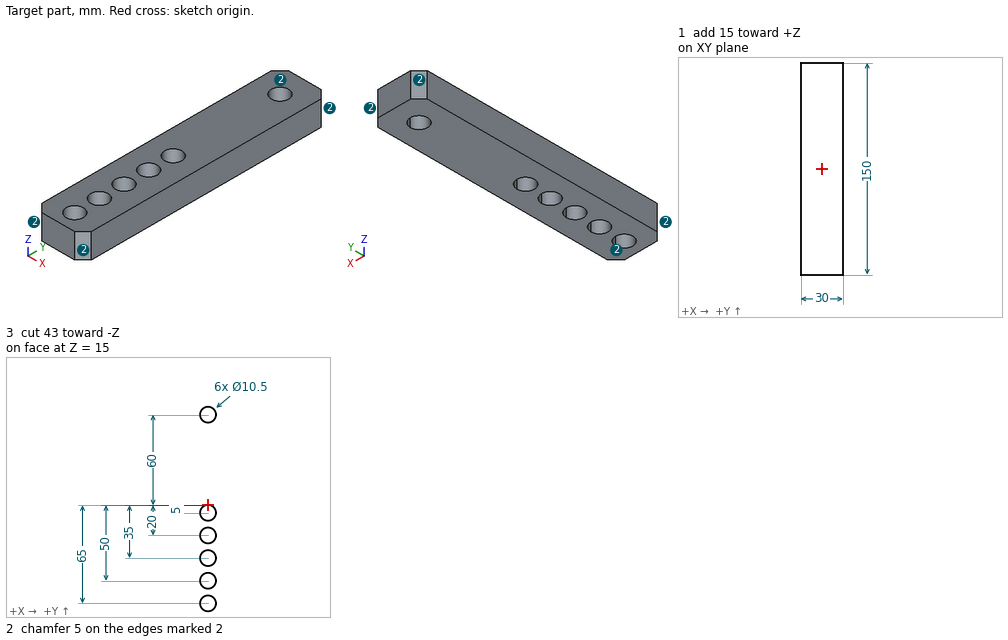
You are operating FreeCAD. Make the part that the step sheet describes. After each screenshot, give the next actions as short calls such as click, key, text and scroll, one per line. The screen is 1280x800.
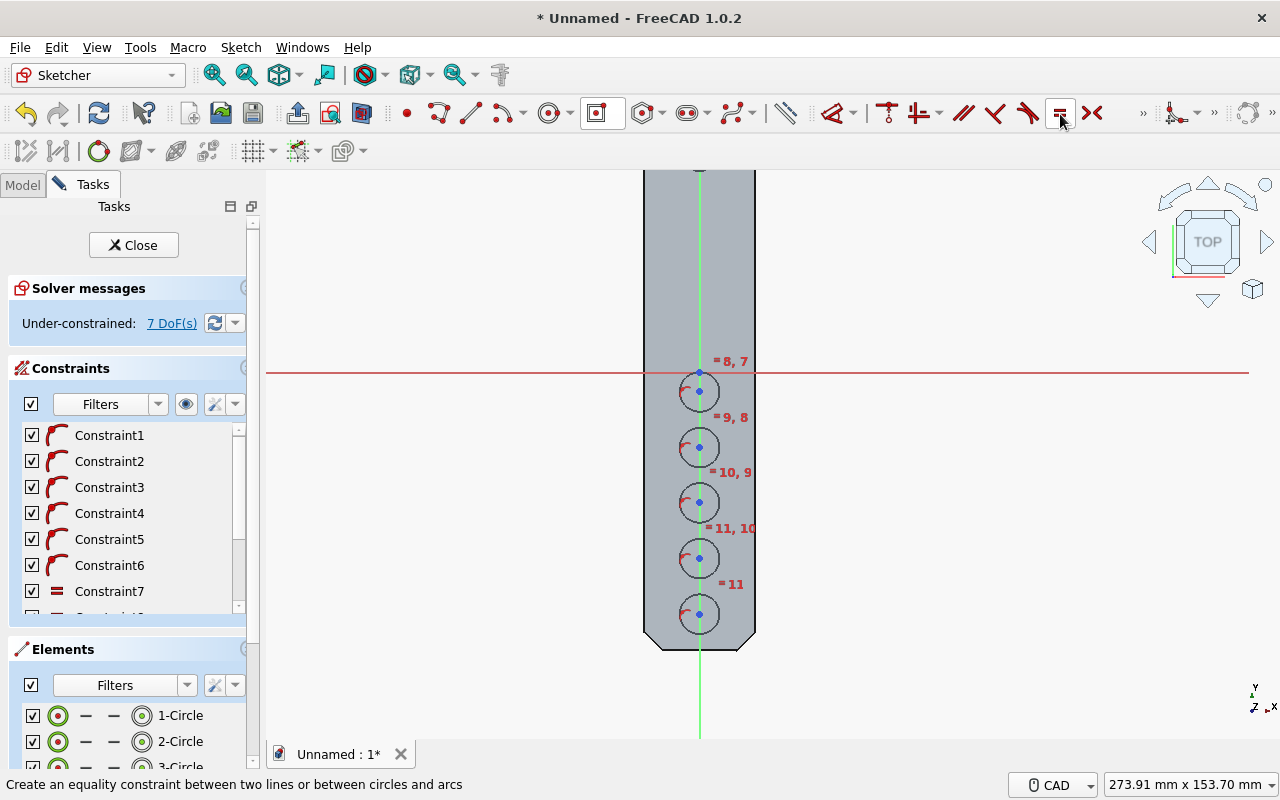
scroll(714, 602, down, 2)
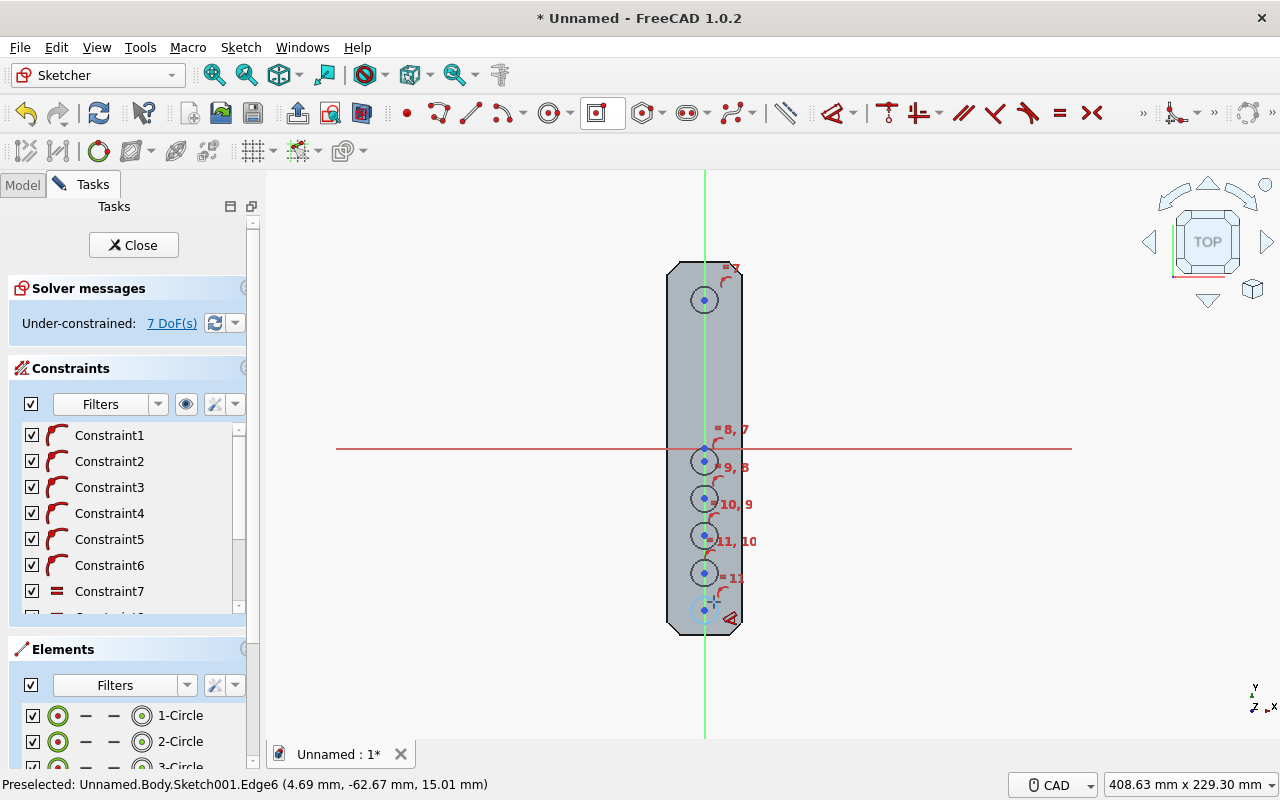
scroll(714, 291, up, 3)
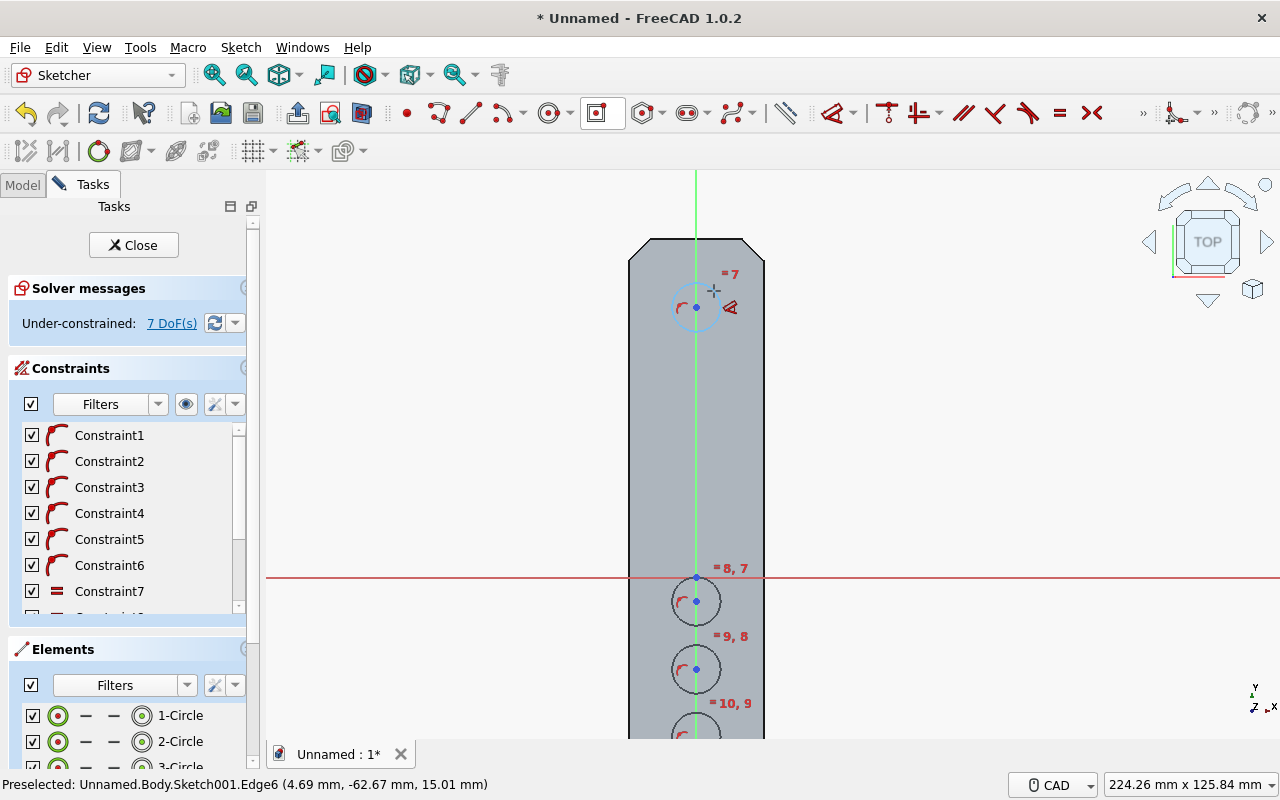
click(713, 290)
click(735, 267)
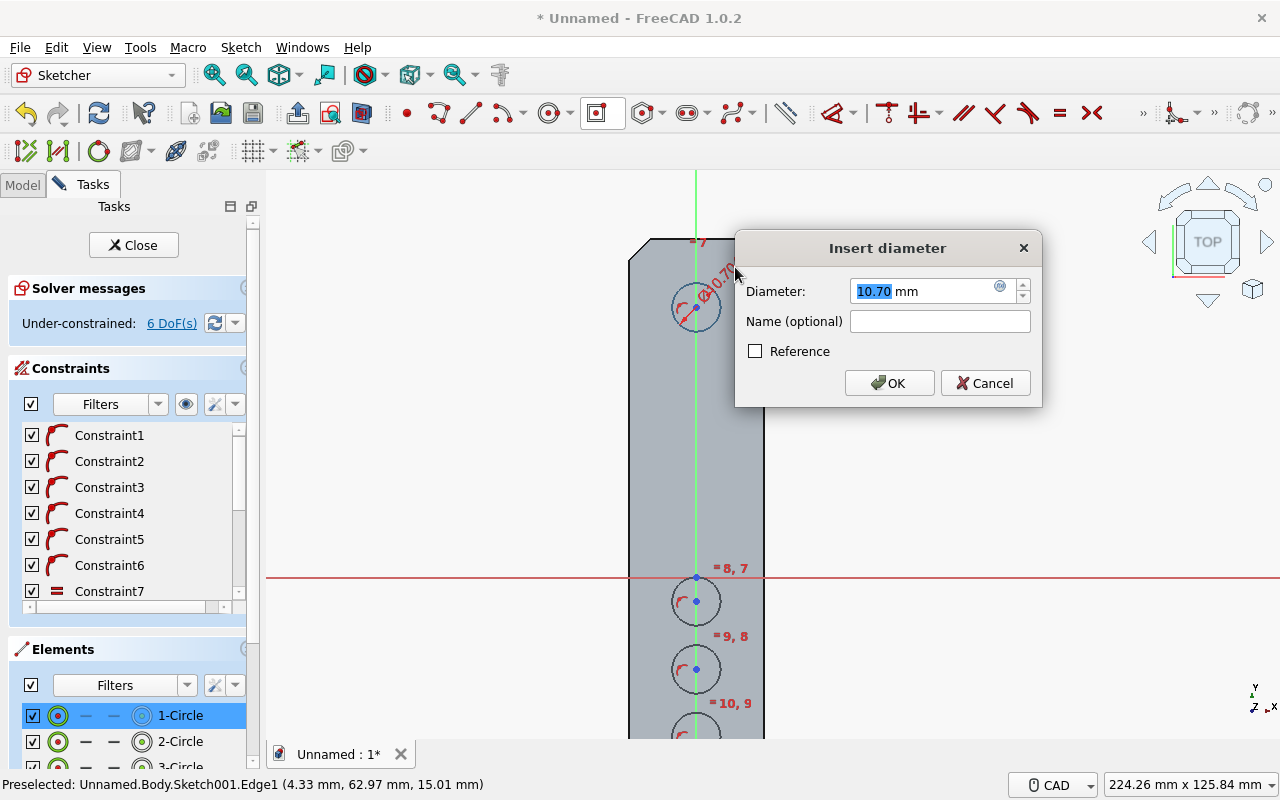
text(10.5)
key(Return)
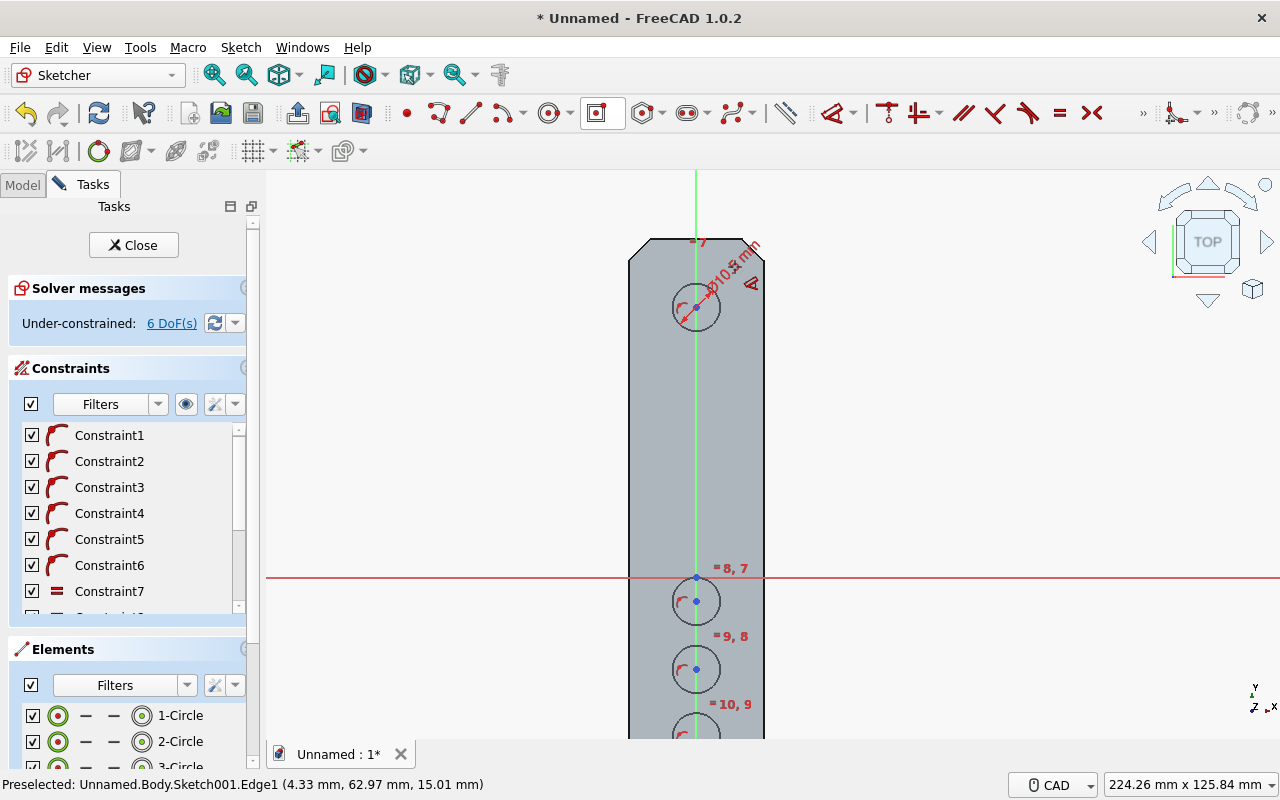
scroll(696, 601, up, 3)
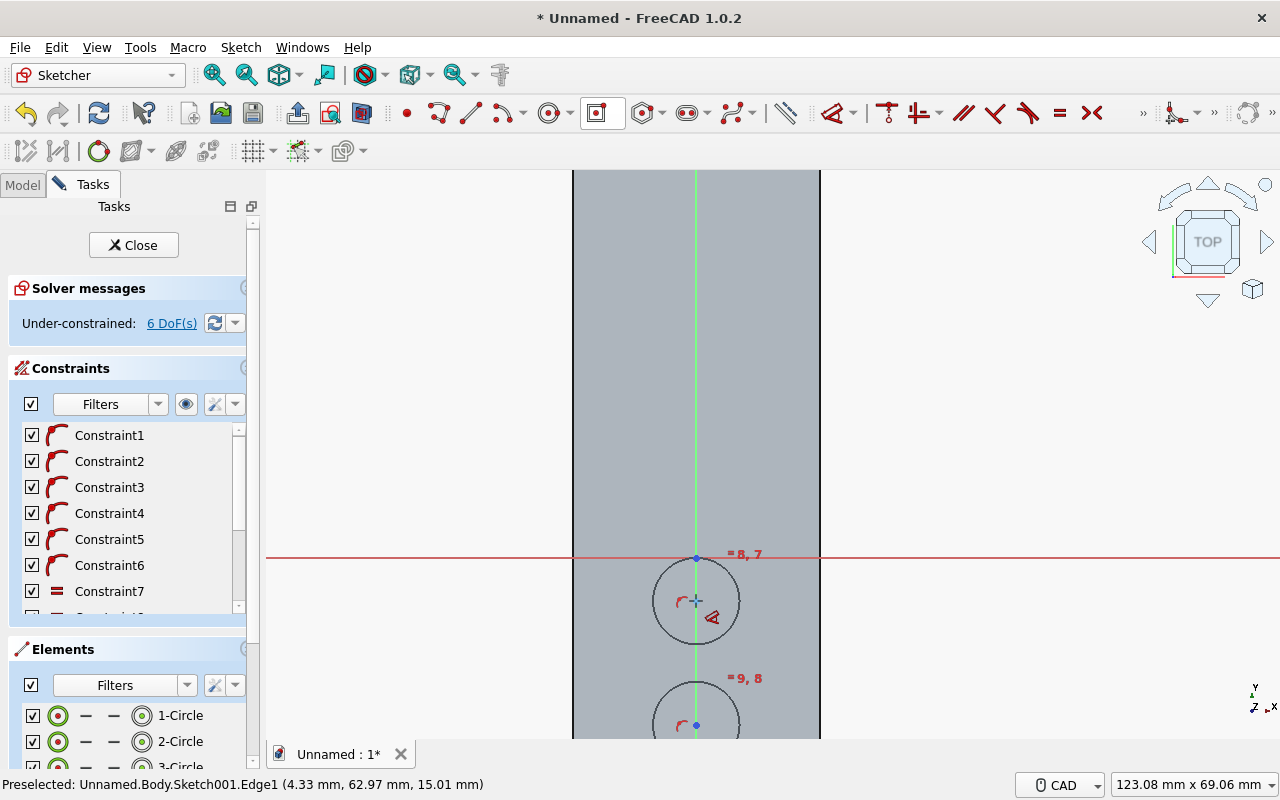
click(696, 601)
click(754, 580)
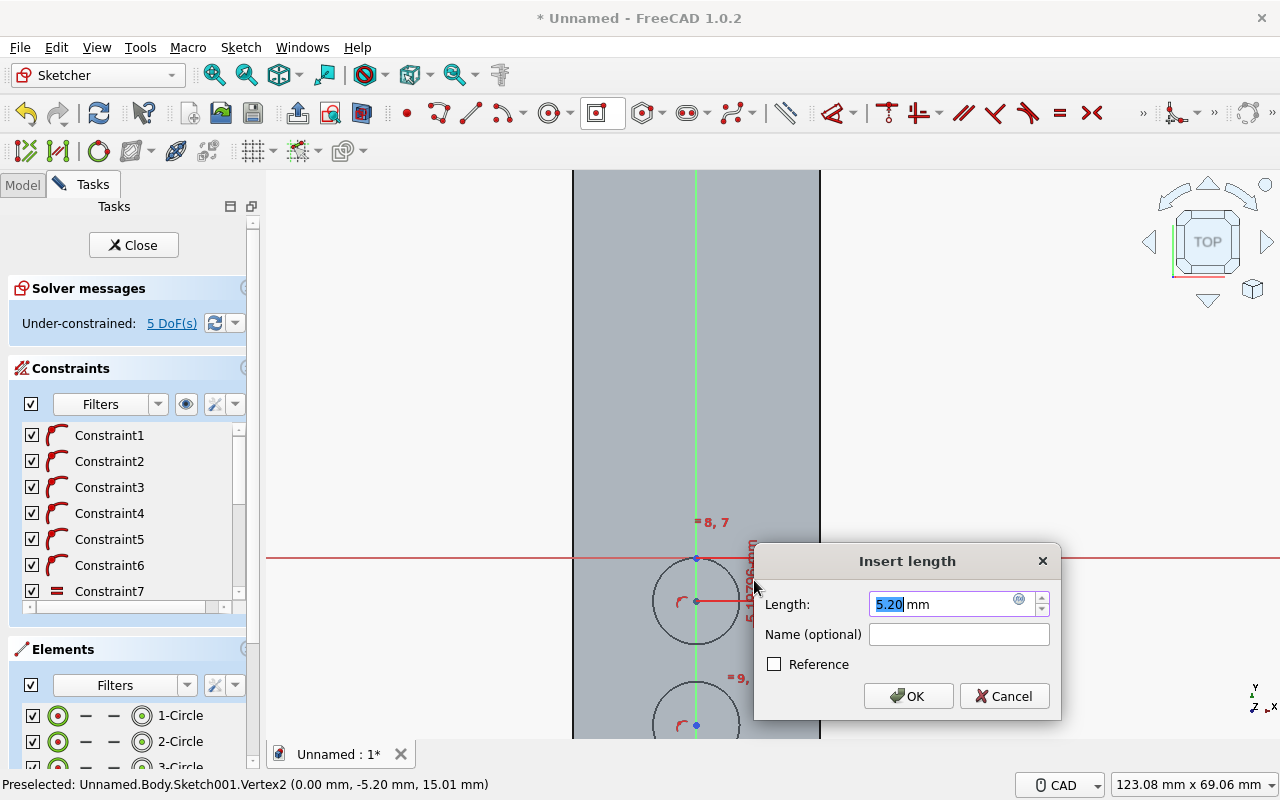
text(5)
key(Return)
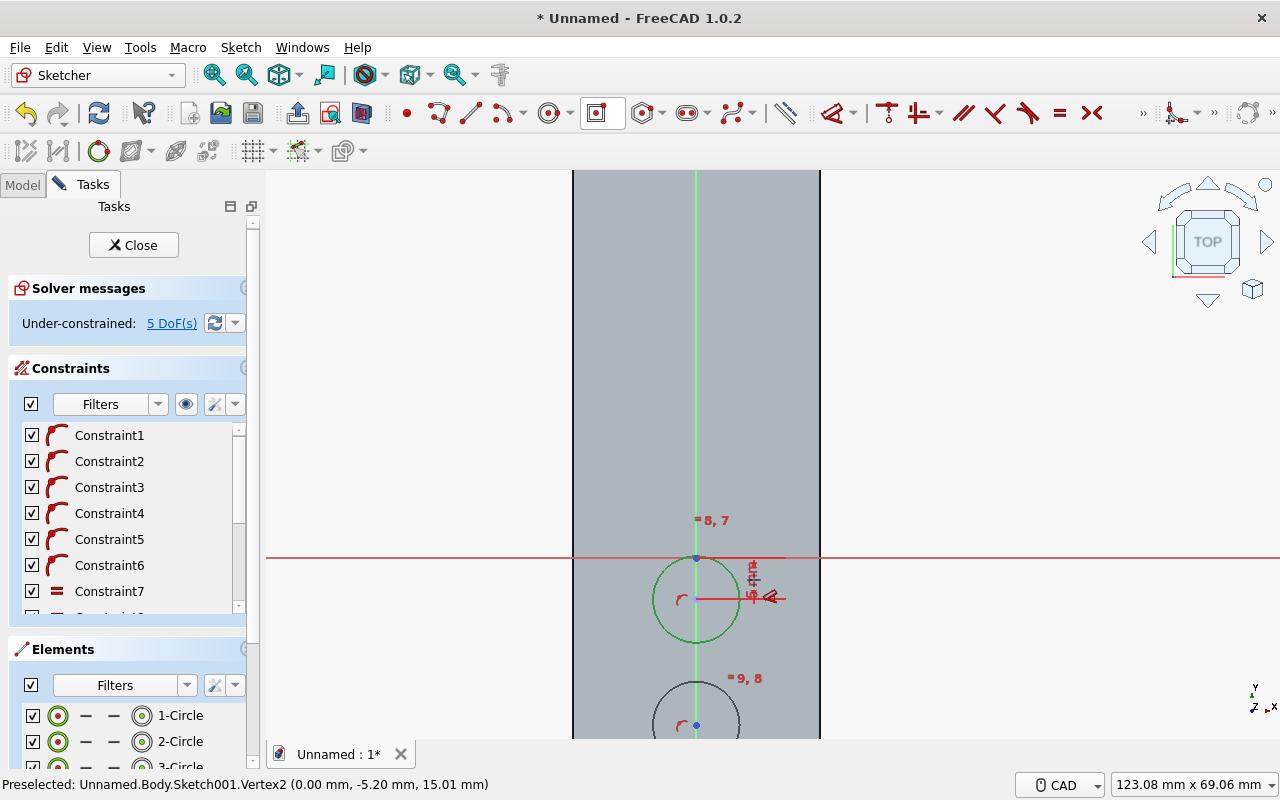
scroll(708, 401, down, 6)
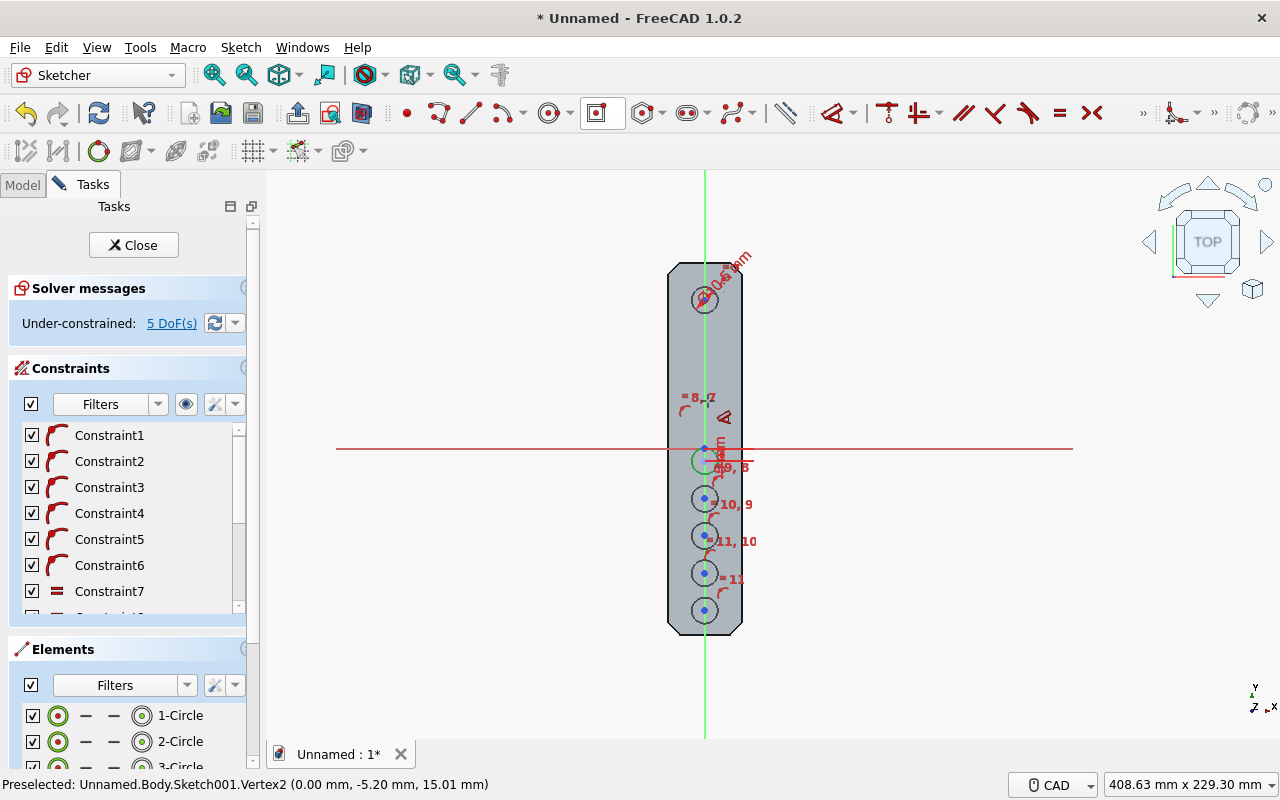
click(705, 300)
click(739, 374)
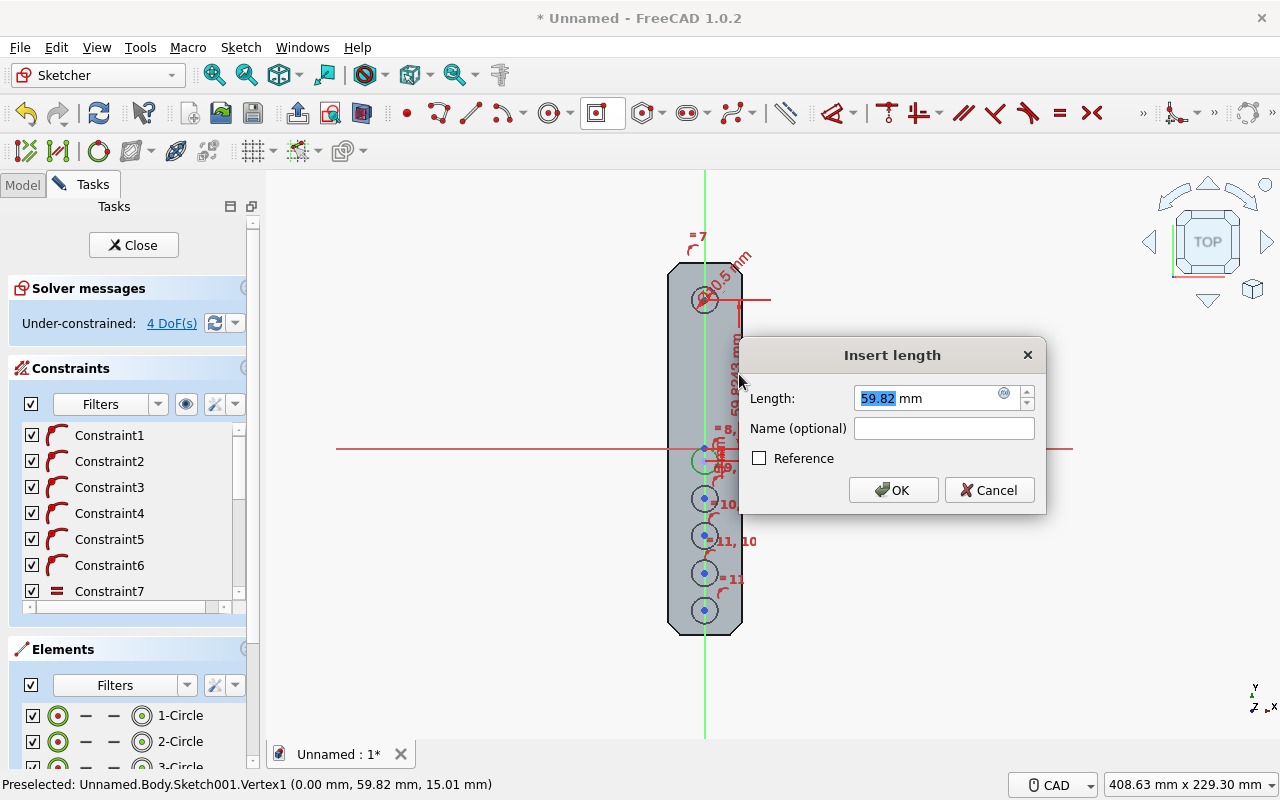
text(60)
key(Return)